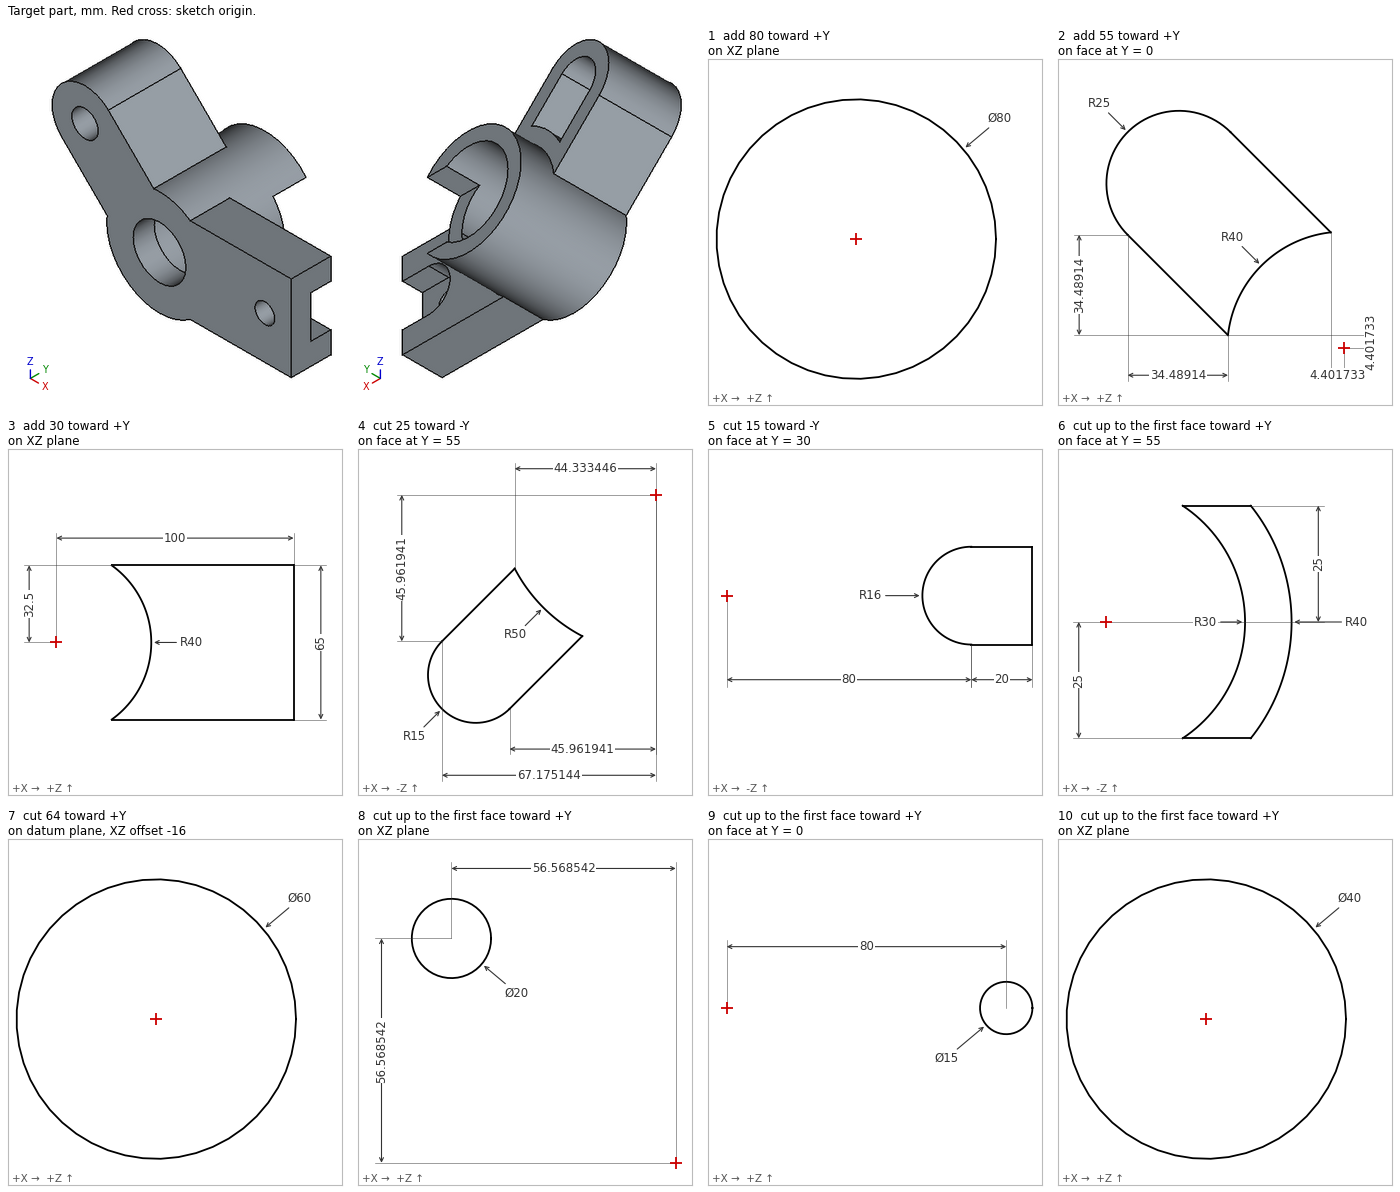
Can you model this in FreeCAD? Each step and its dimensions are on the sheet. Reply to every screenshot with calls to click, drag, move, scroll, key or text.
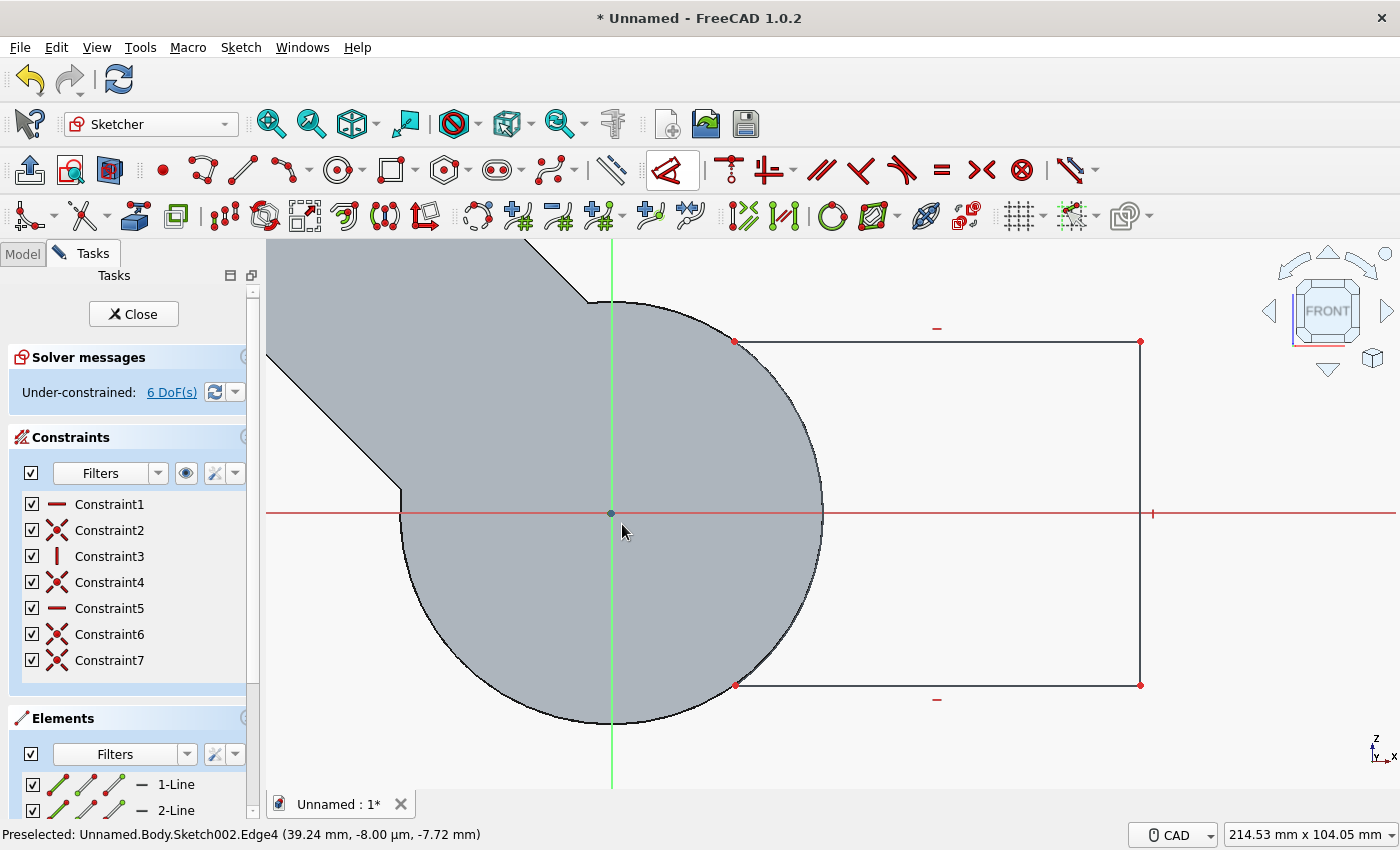
click(730, 170)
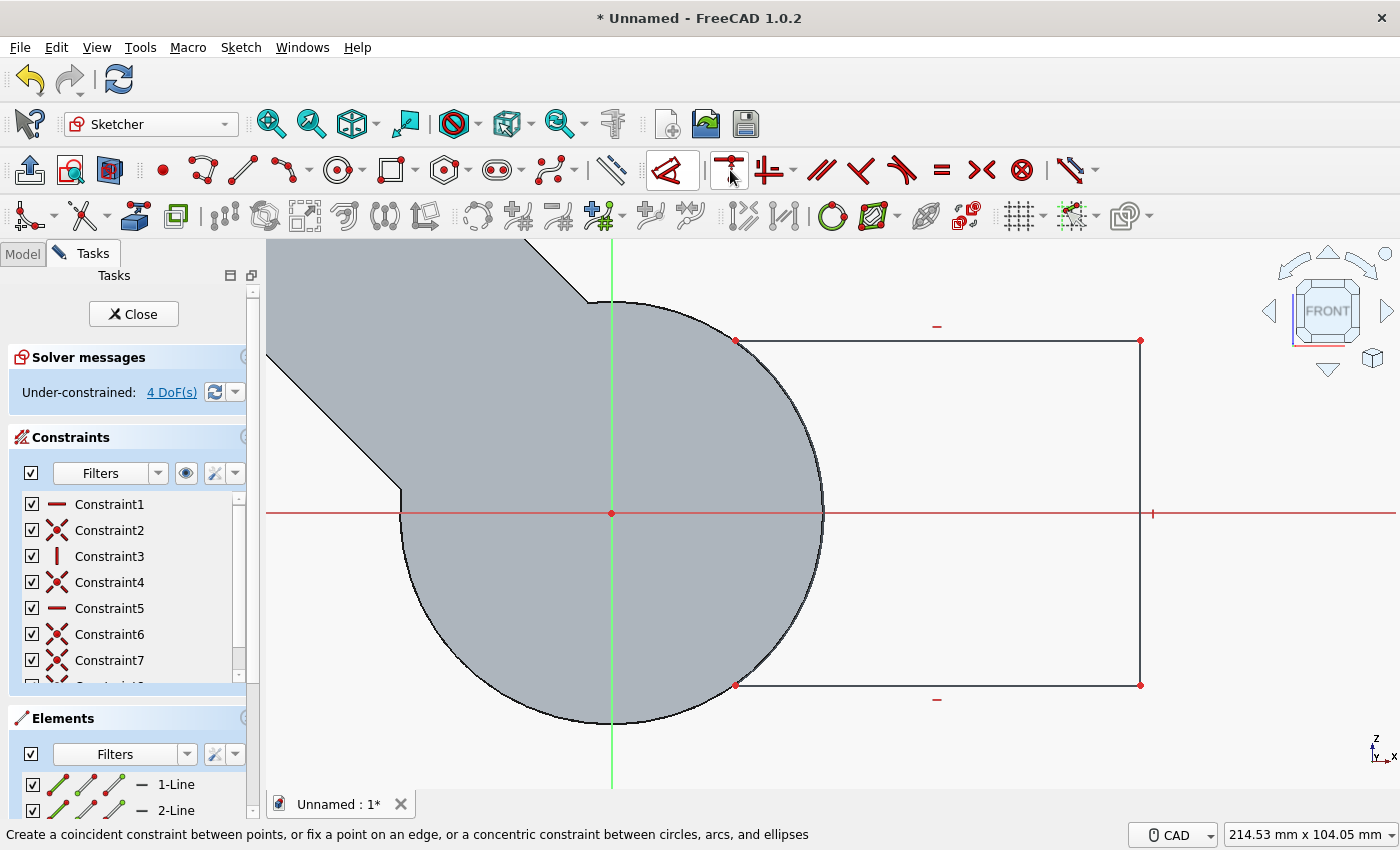
click(809, 592)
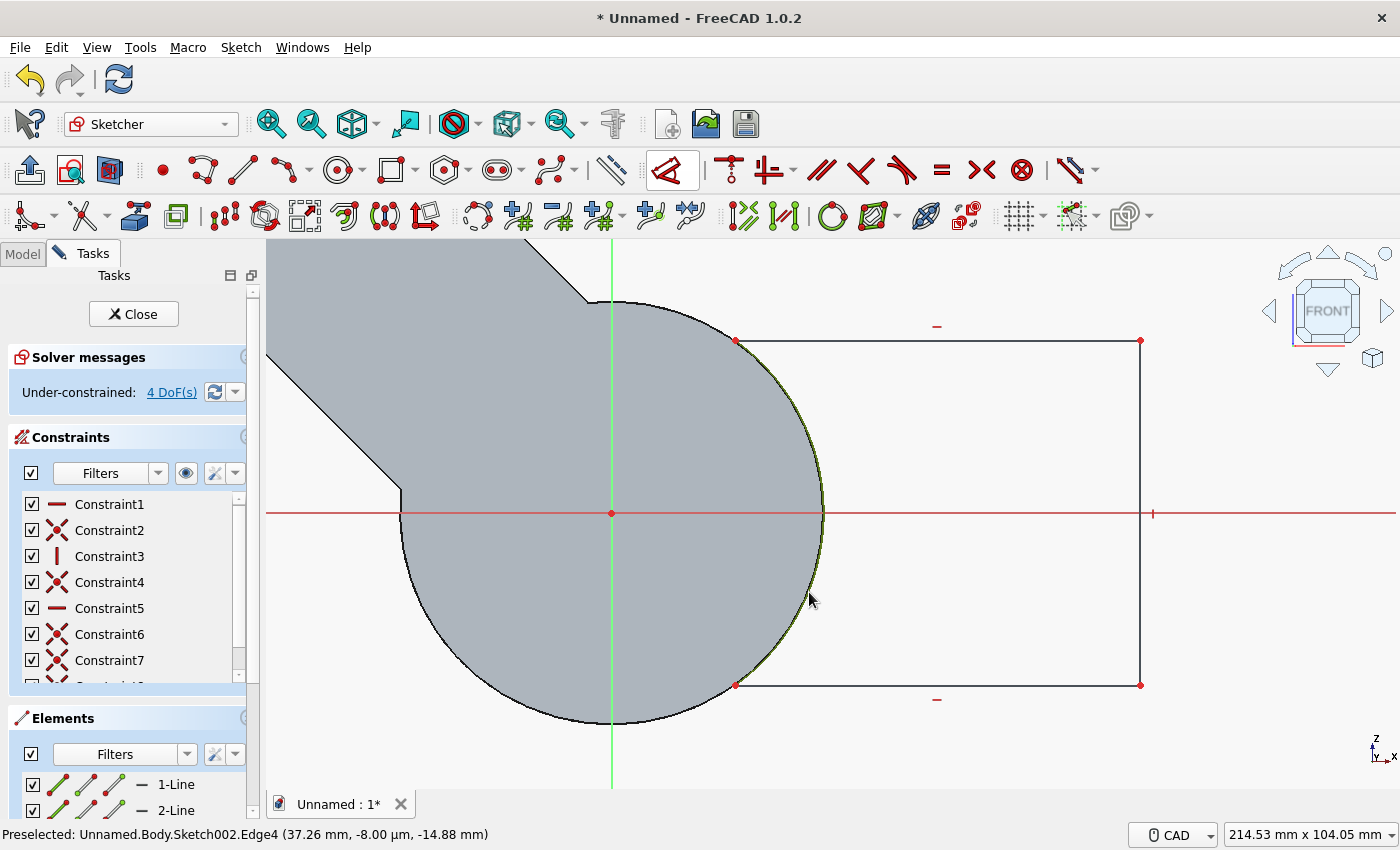
key(k)
key(r)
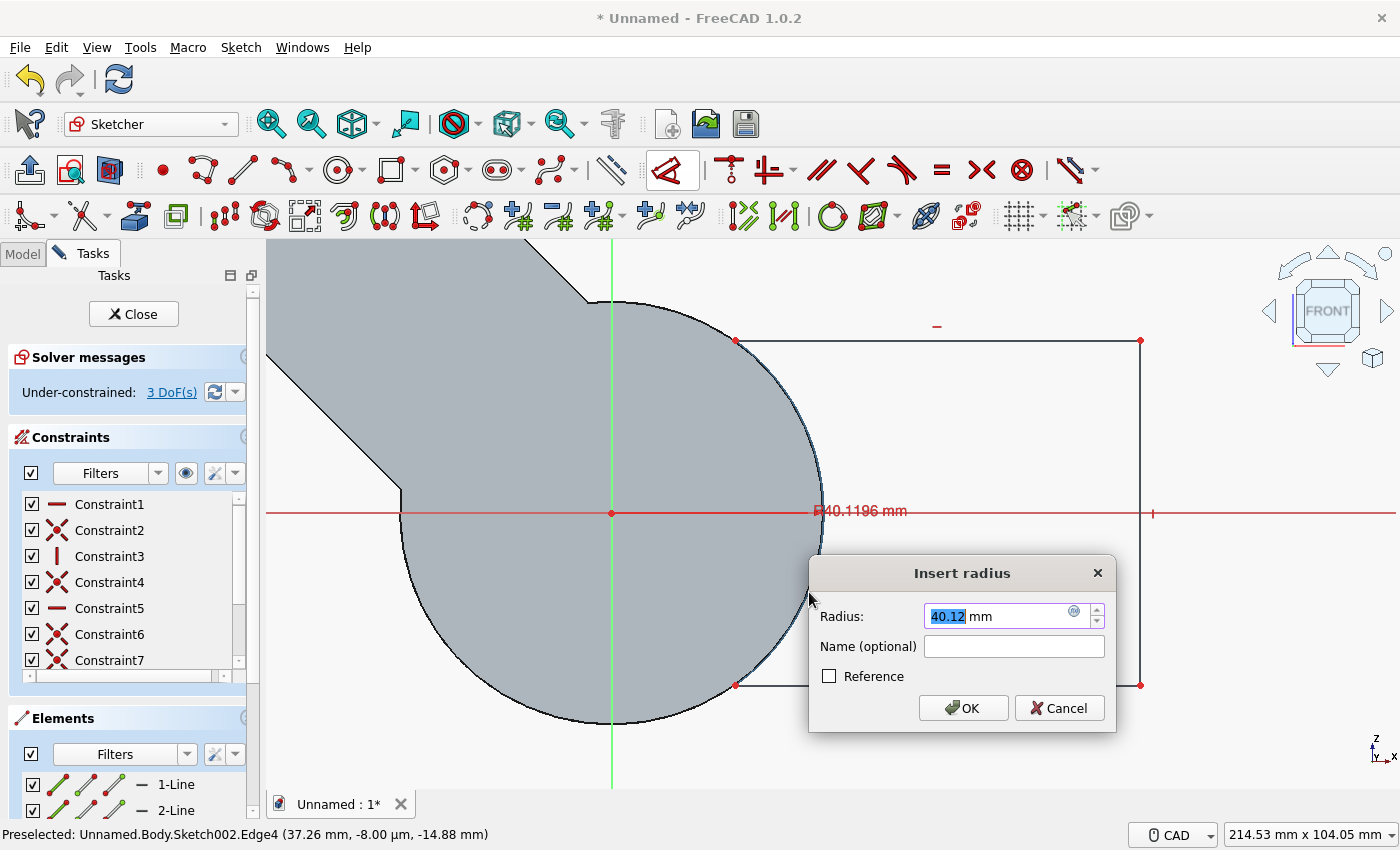
text(40)
key(Return)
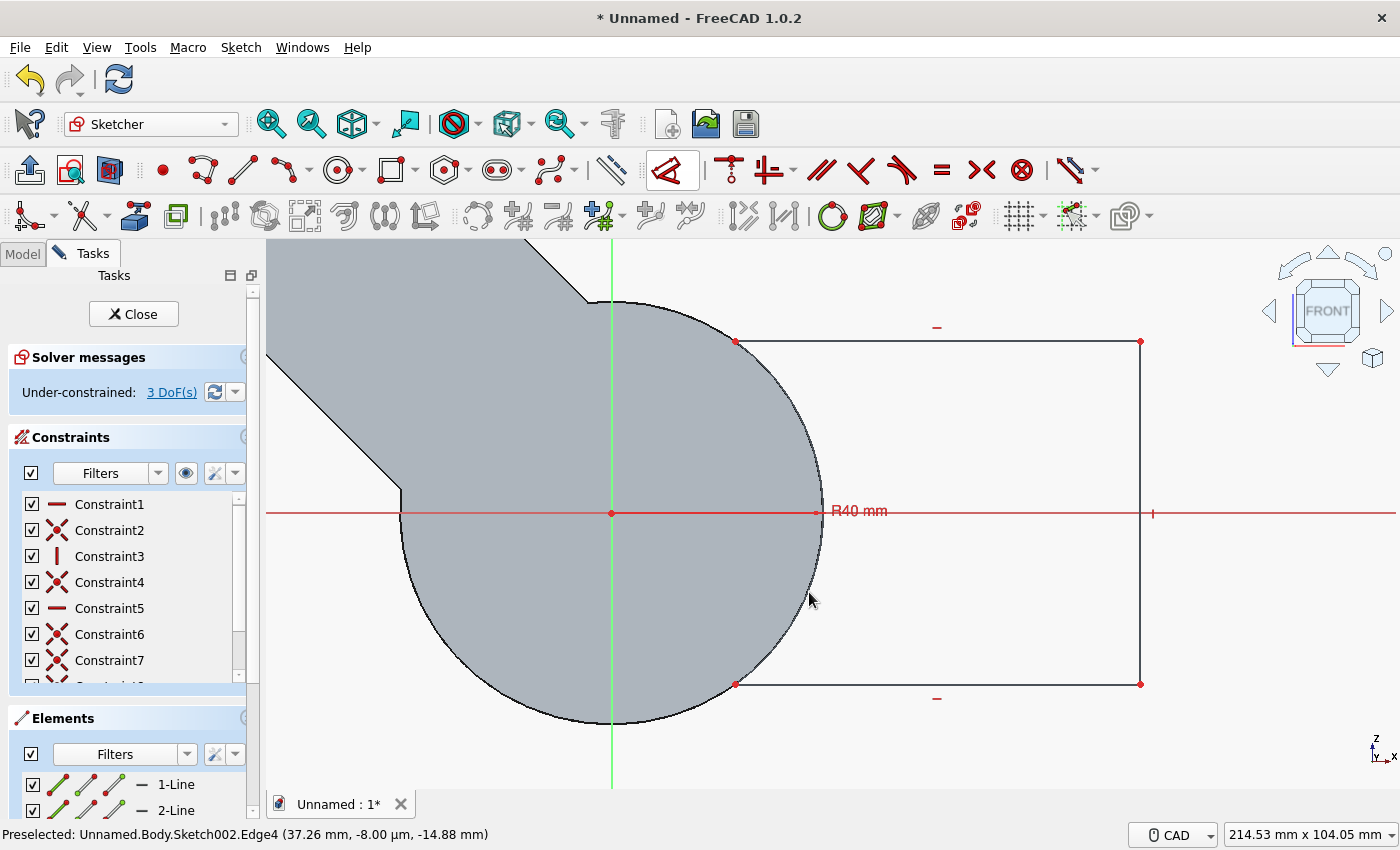
click(1140, 444)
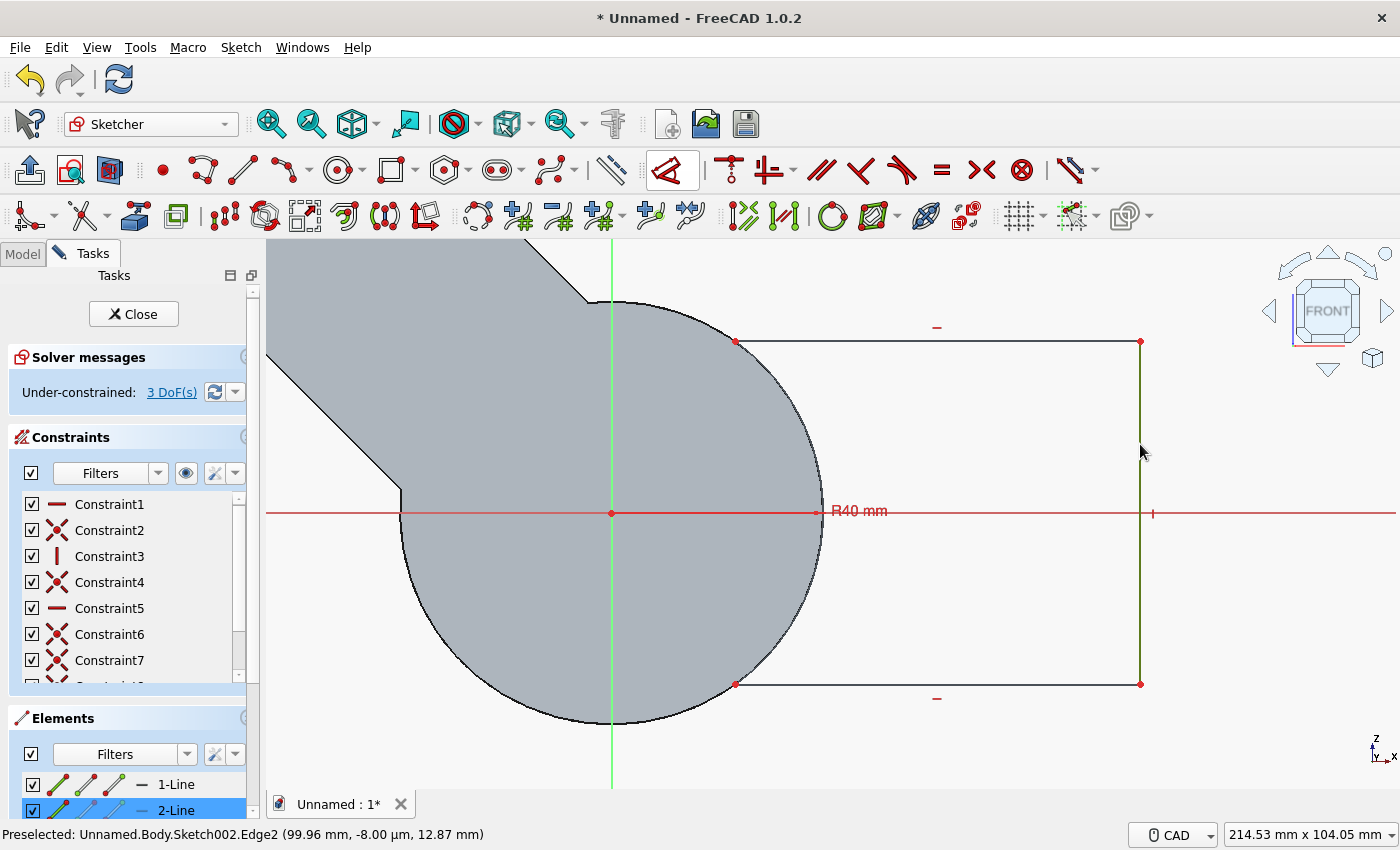
click(694, 170)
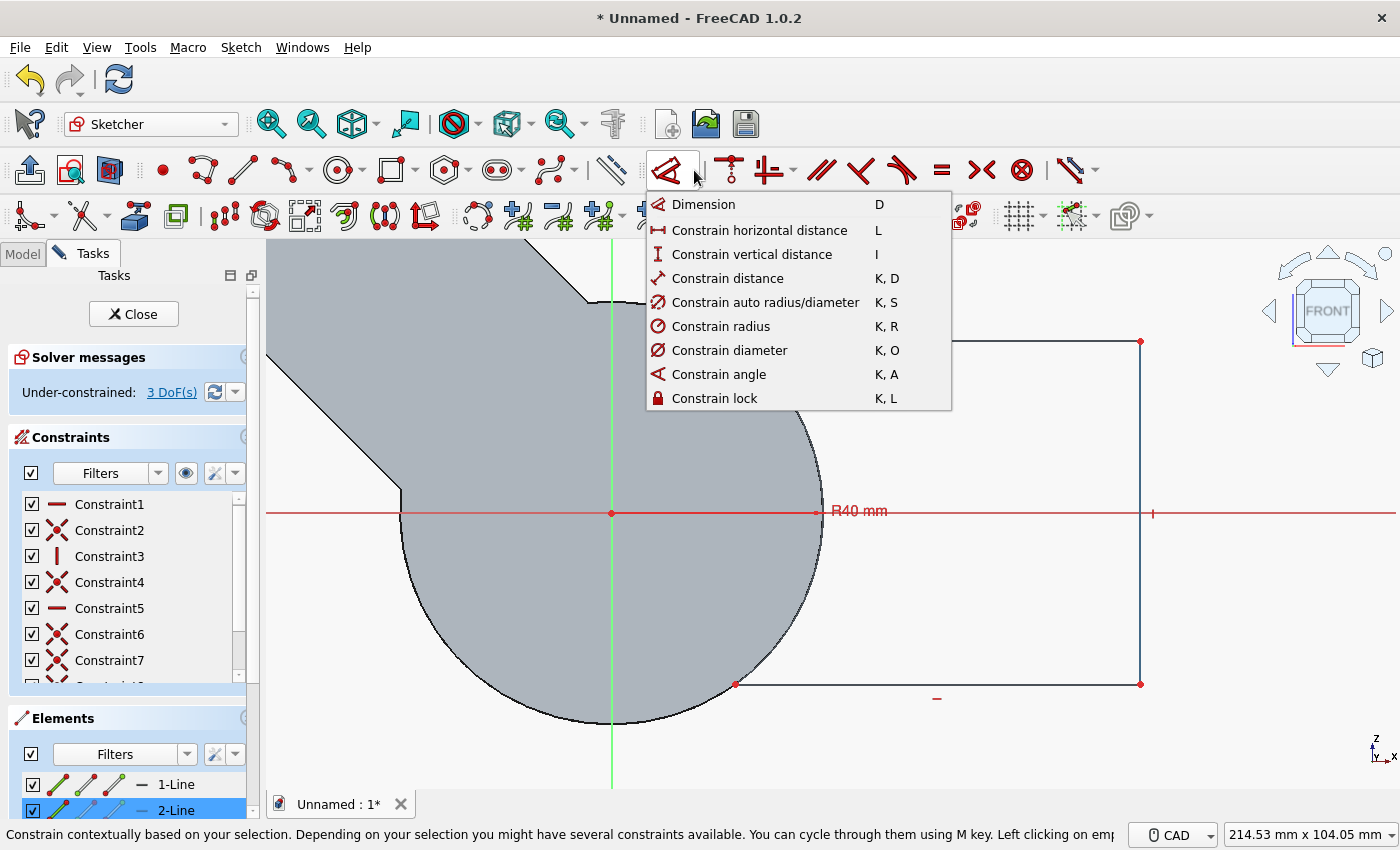
click(799, 254)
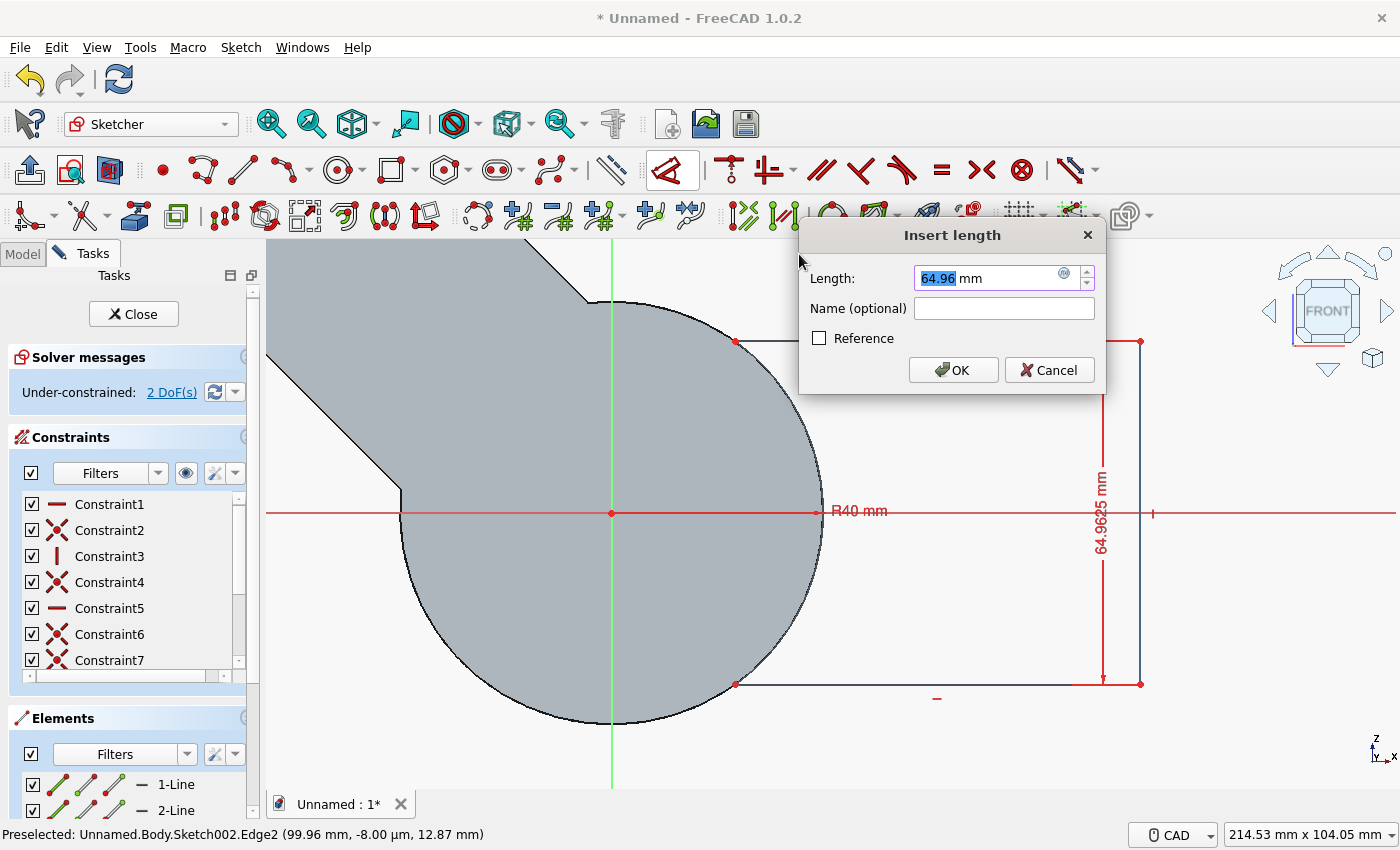
text(65)
key(Return)